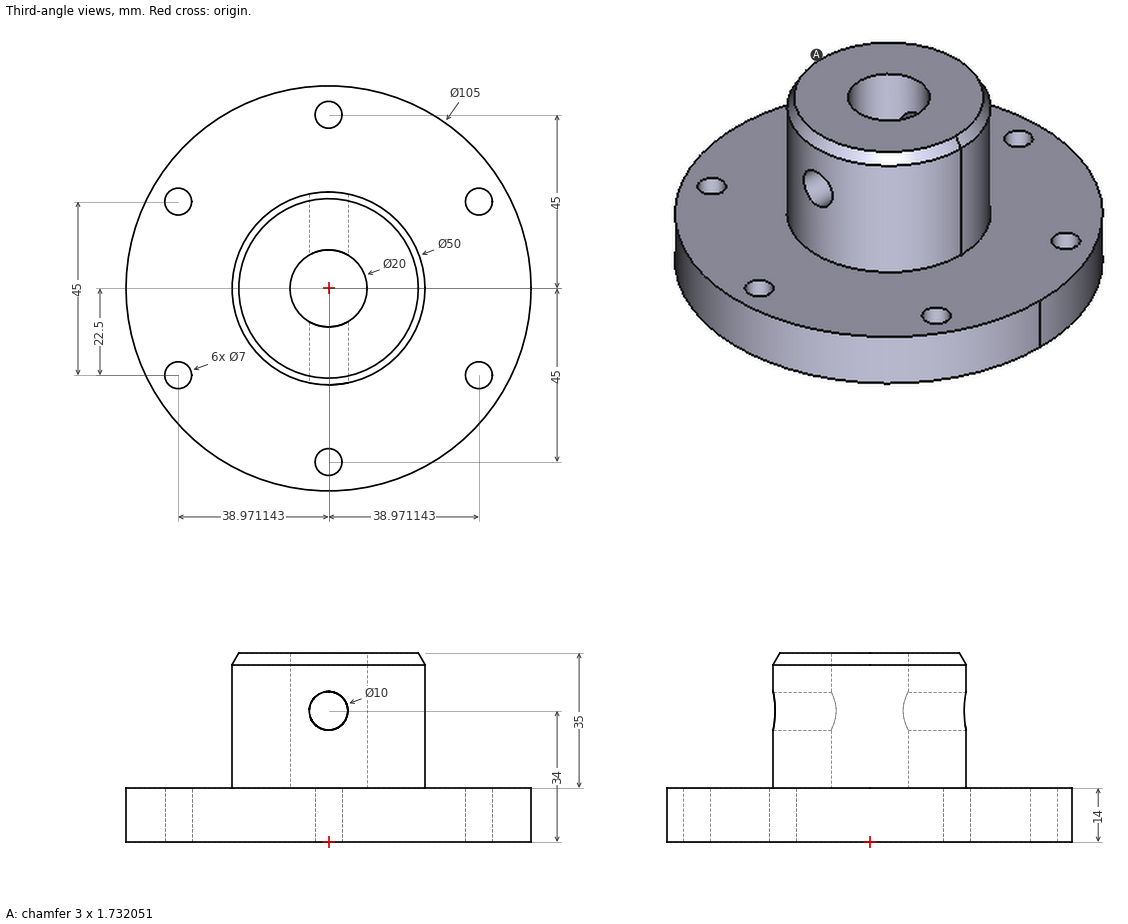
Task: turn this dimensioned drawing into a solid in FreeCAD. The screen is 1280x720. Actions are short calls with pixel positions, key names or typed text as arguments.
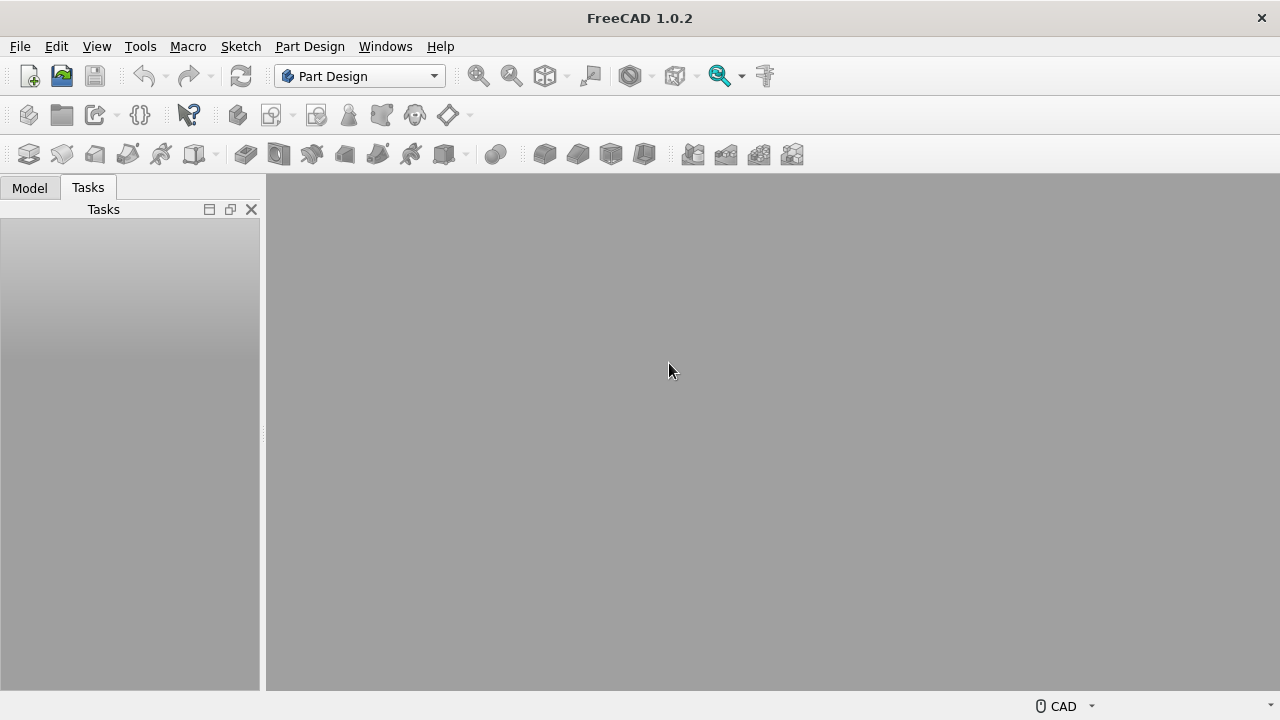
click(29, 76)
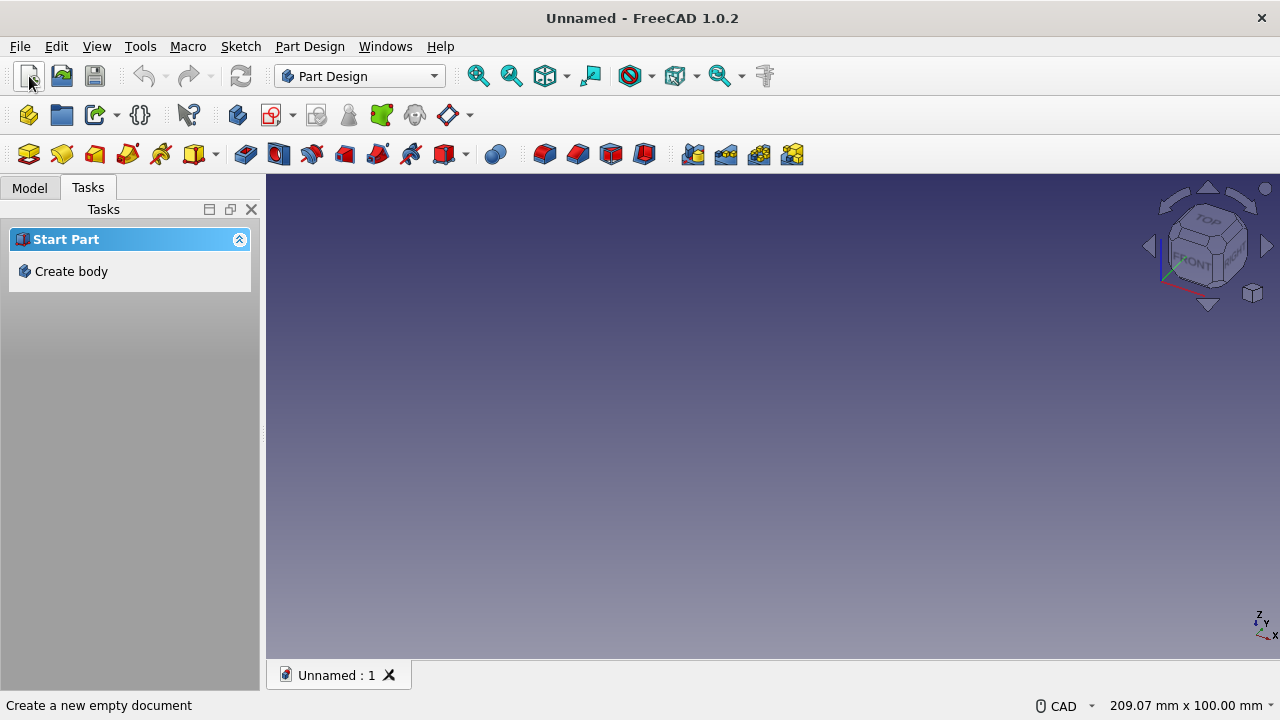
click(270, 116)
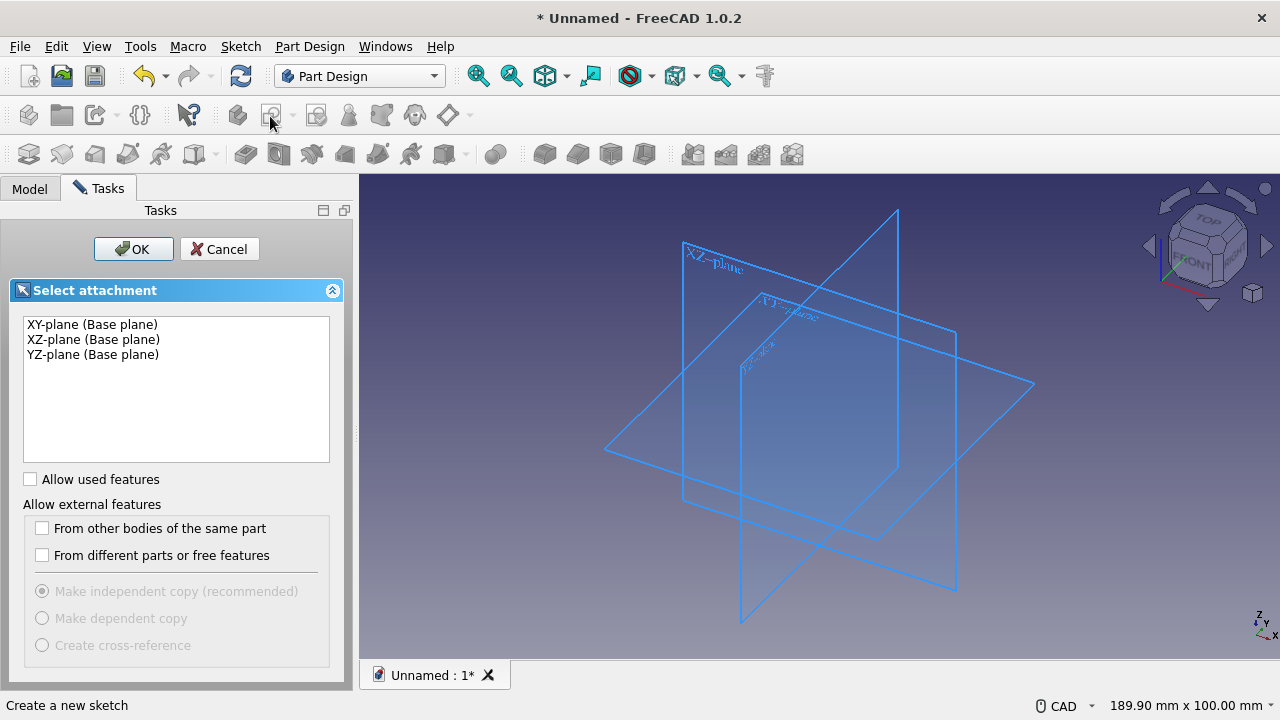
click(84, 324)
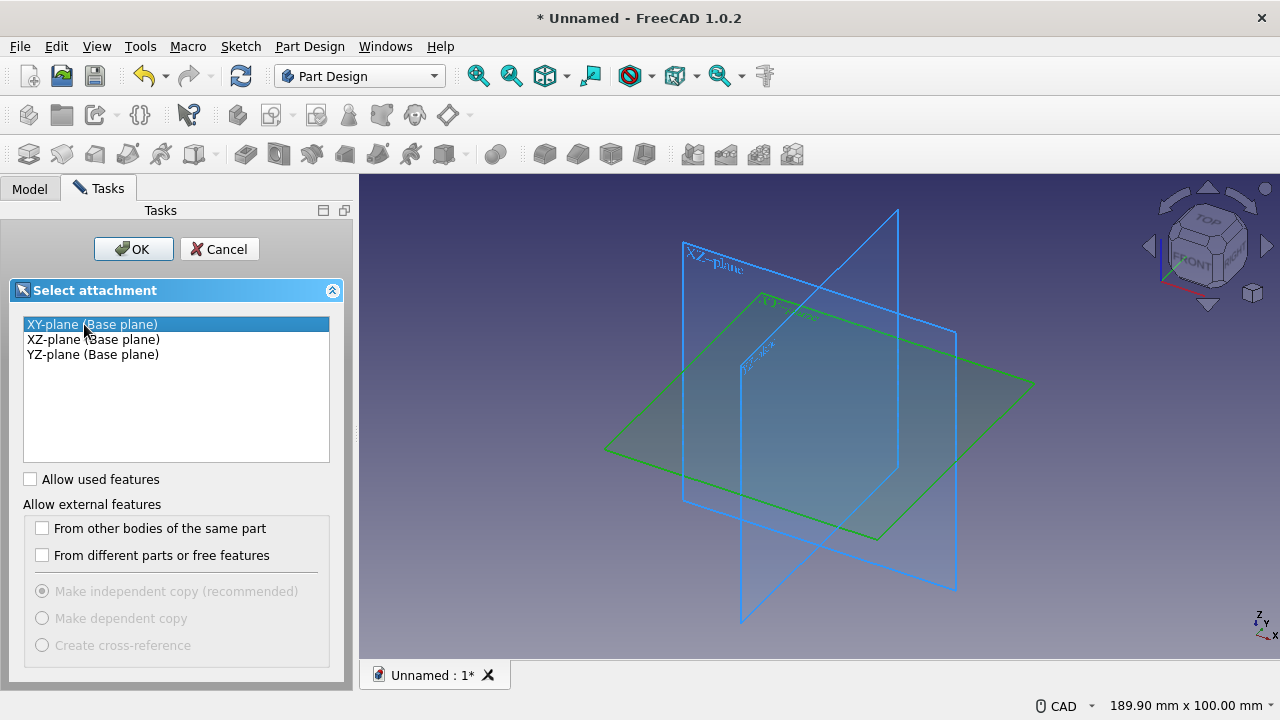
click(134, 249)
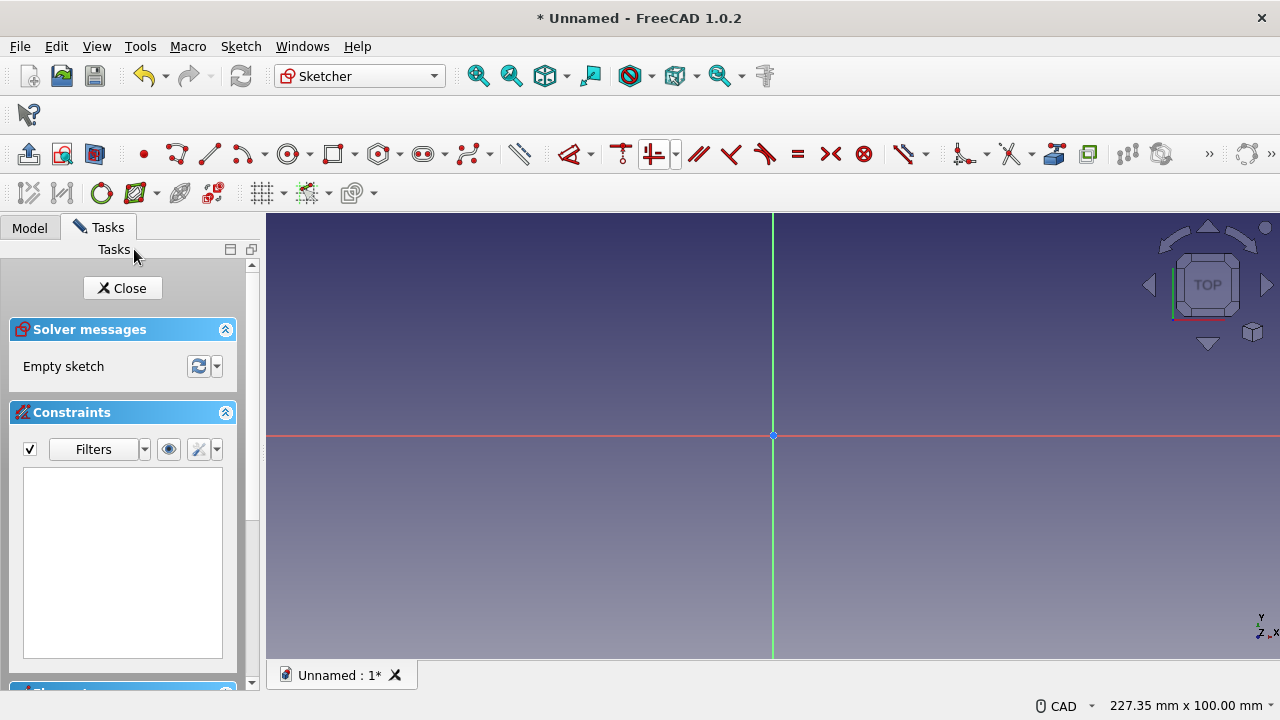
scroll(621, 436, down, 3)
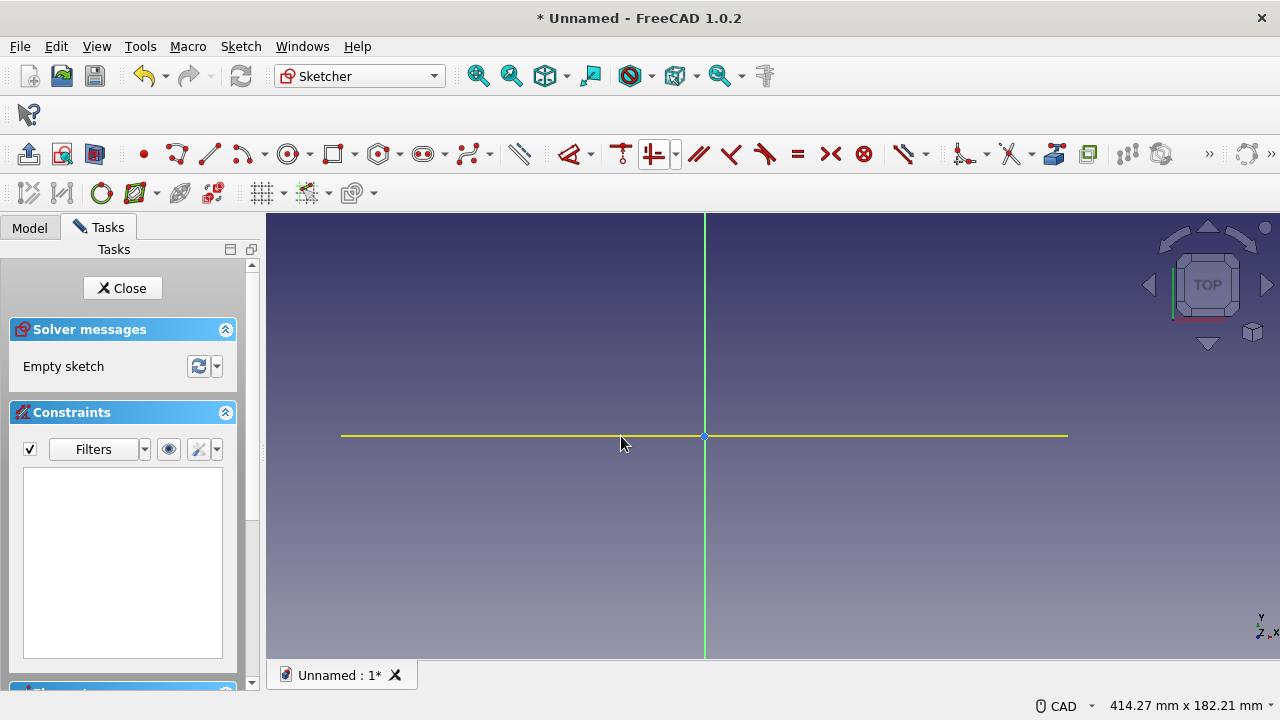
click(288, 154)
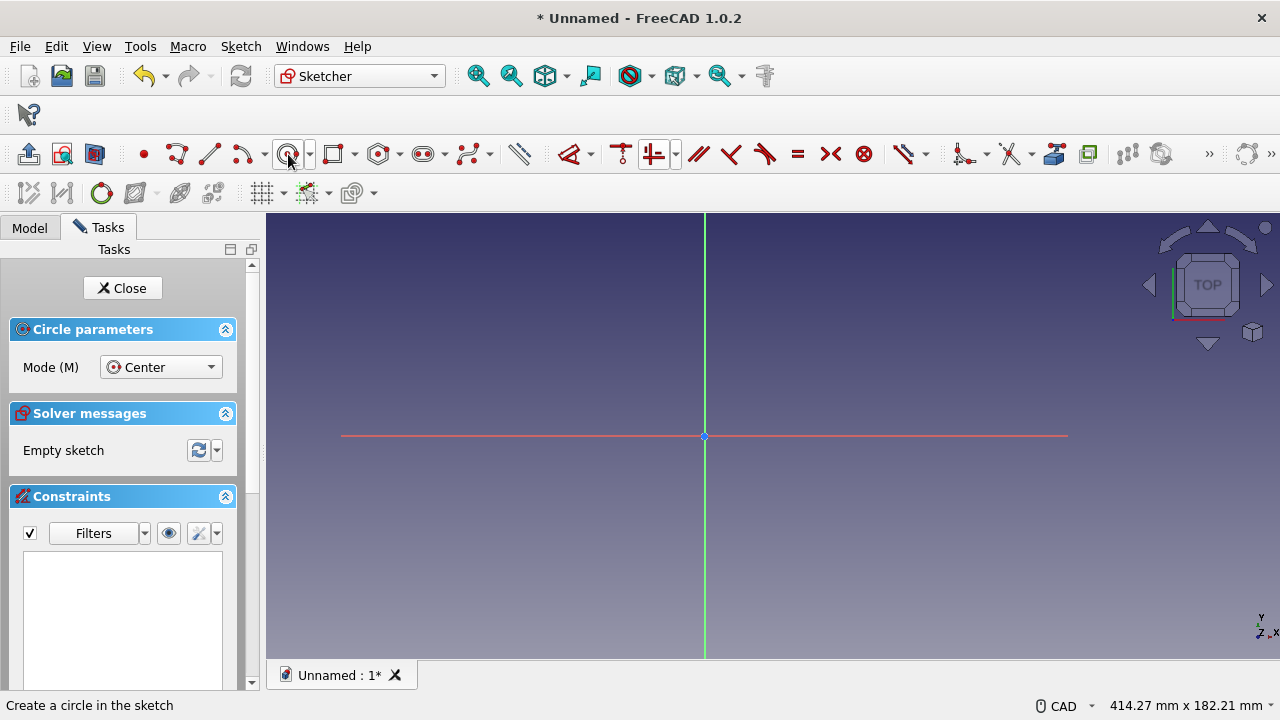
click(705, 436)
click(795, 345)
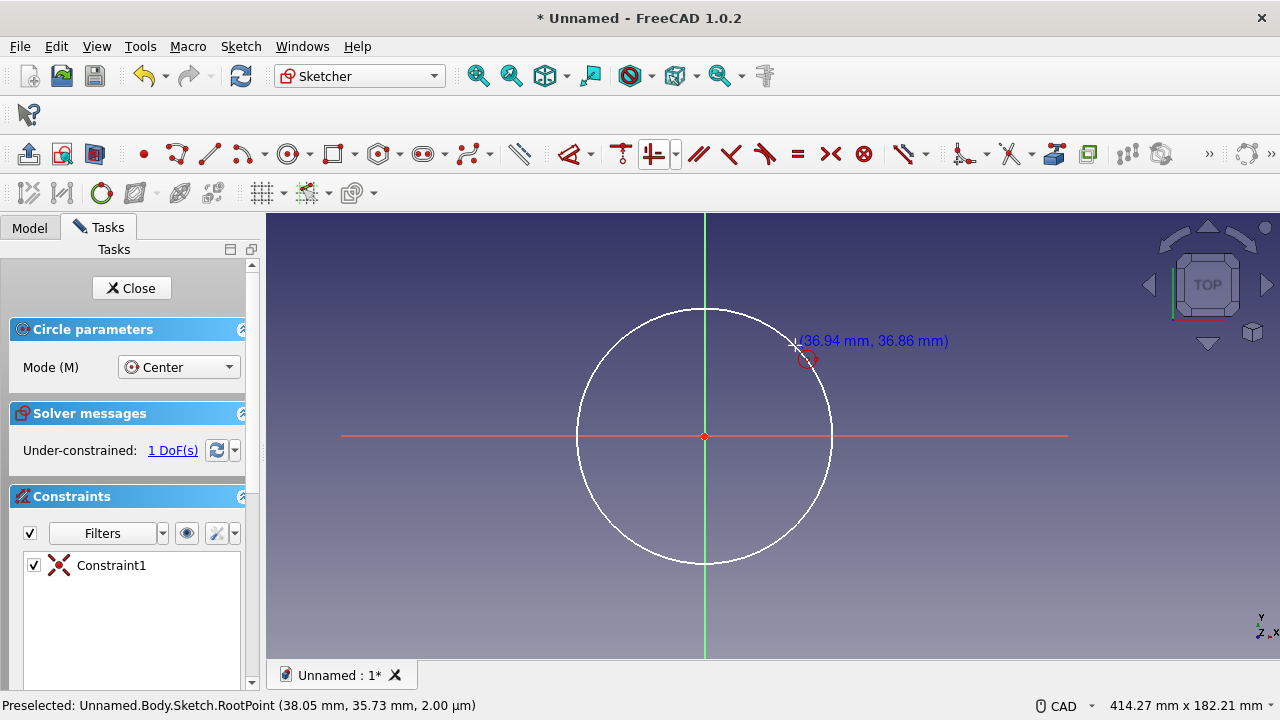
scroll(609, 491, up, 5)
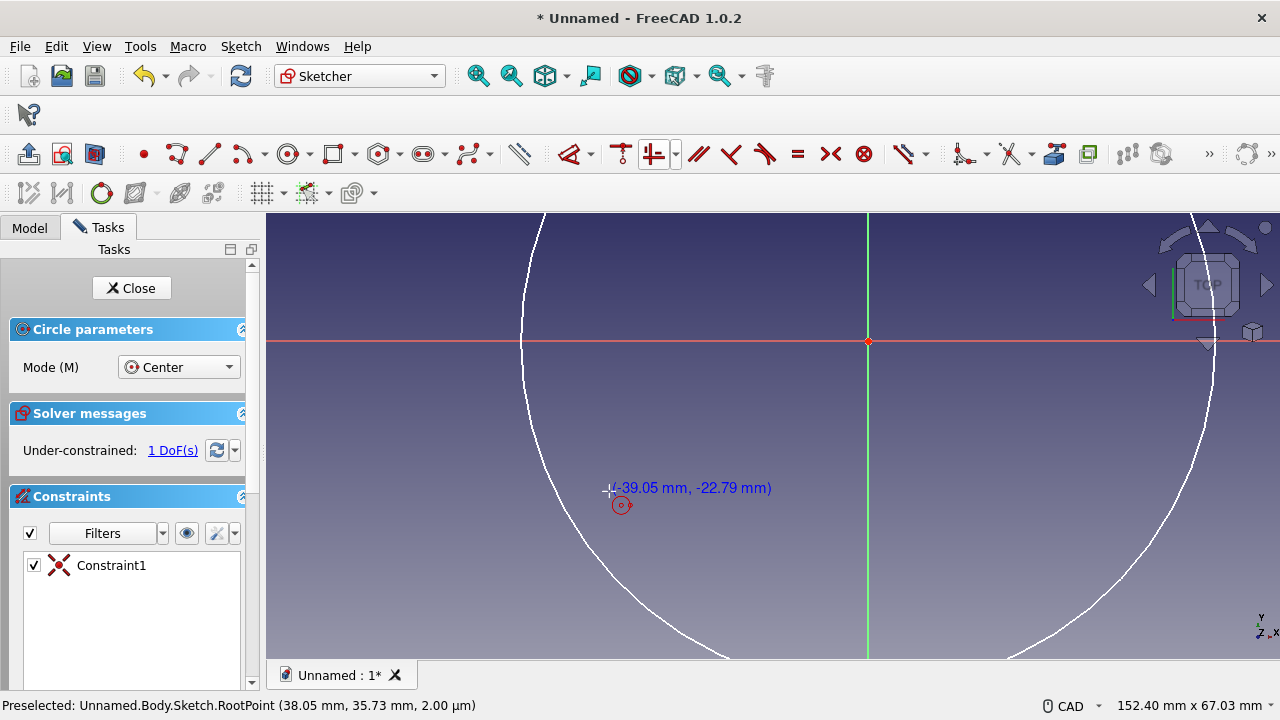
click(609, 491)
click(625, 474)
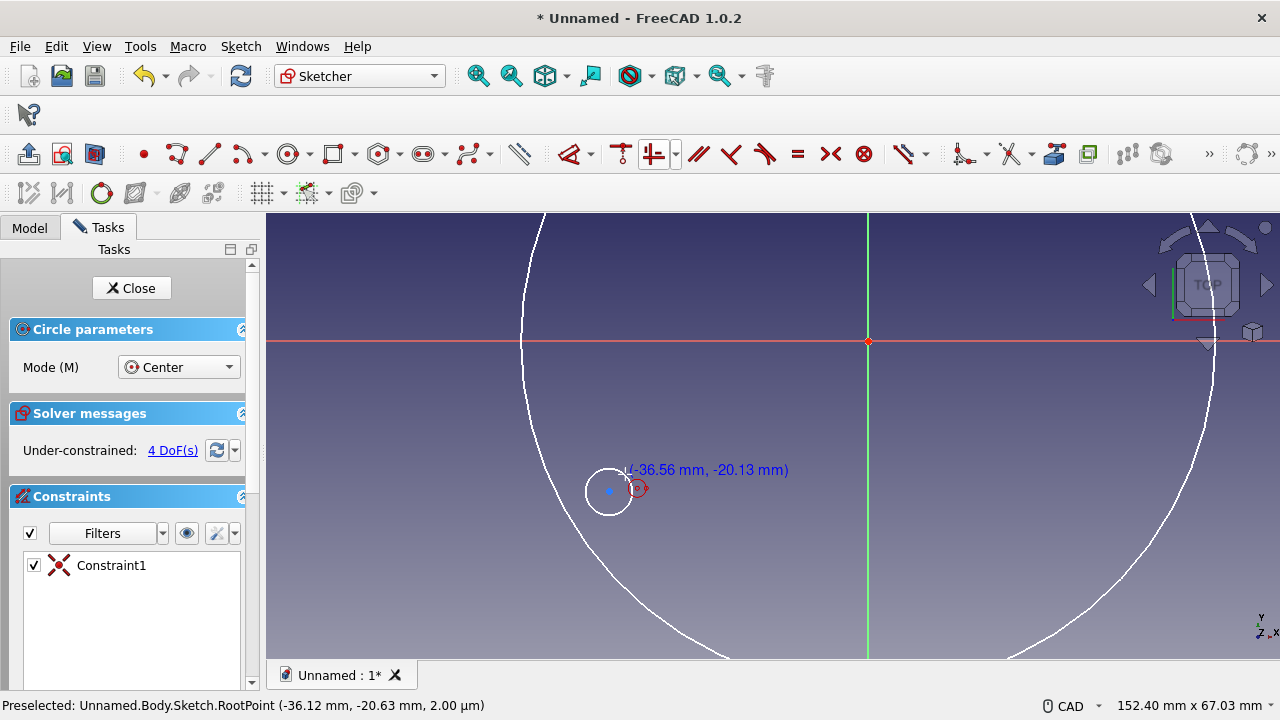
scroll(609, 491, down, 5)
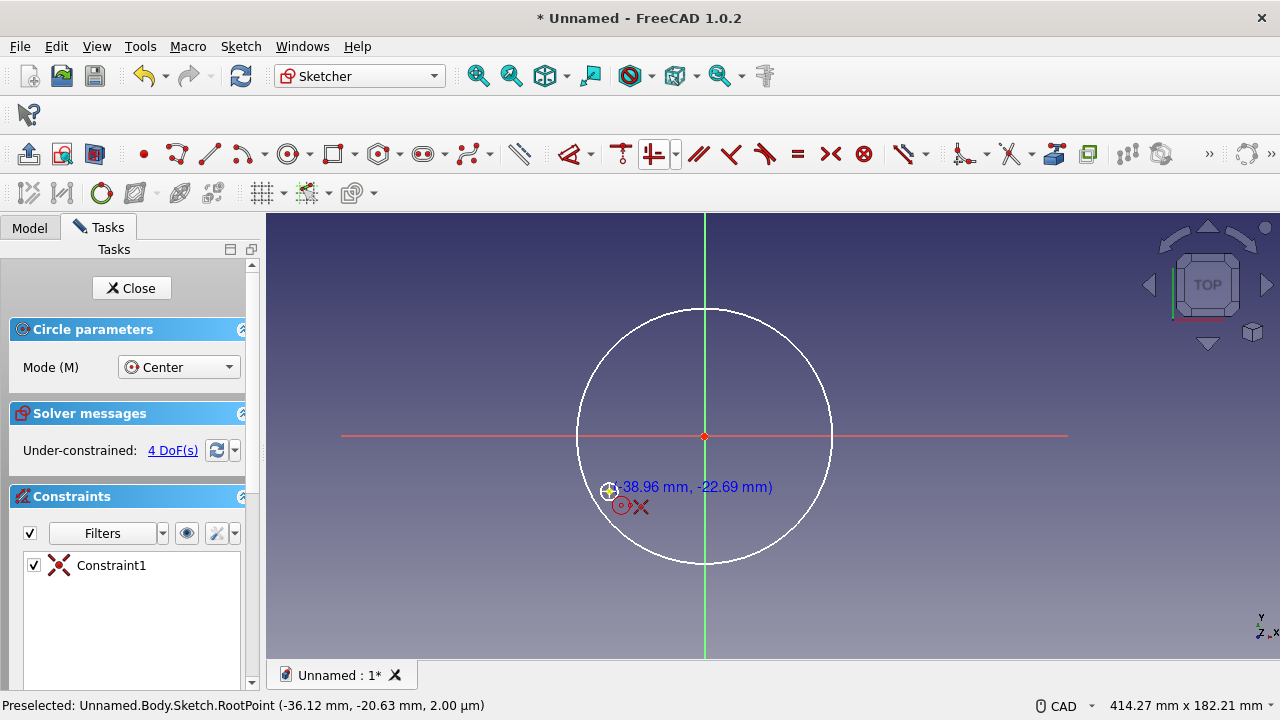
scroll(705, 546, up, 5)